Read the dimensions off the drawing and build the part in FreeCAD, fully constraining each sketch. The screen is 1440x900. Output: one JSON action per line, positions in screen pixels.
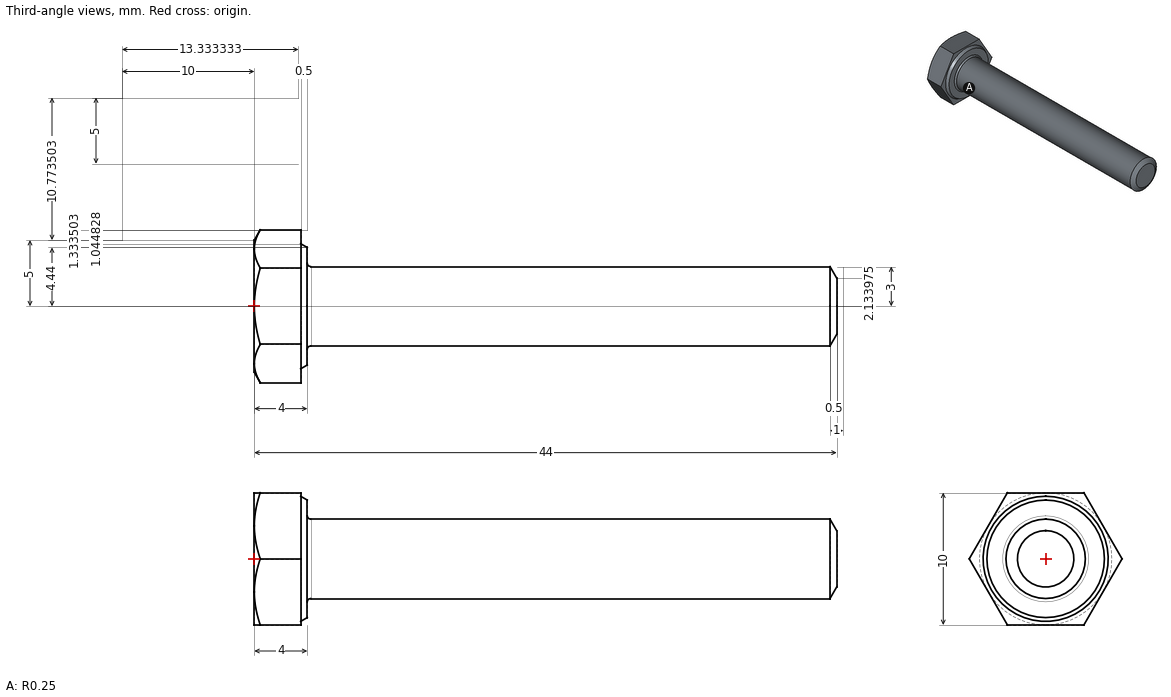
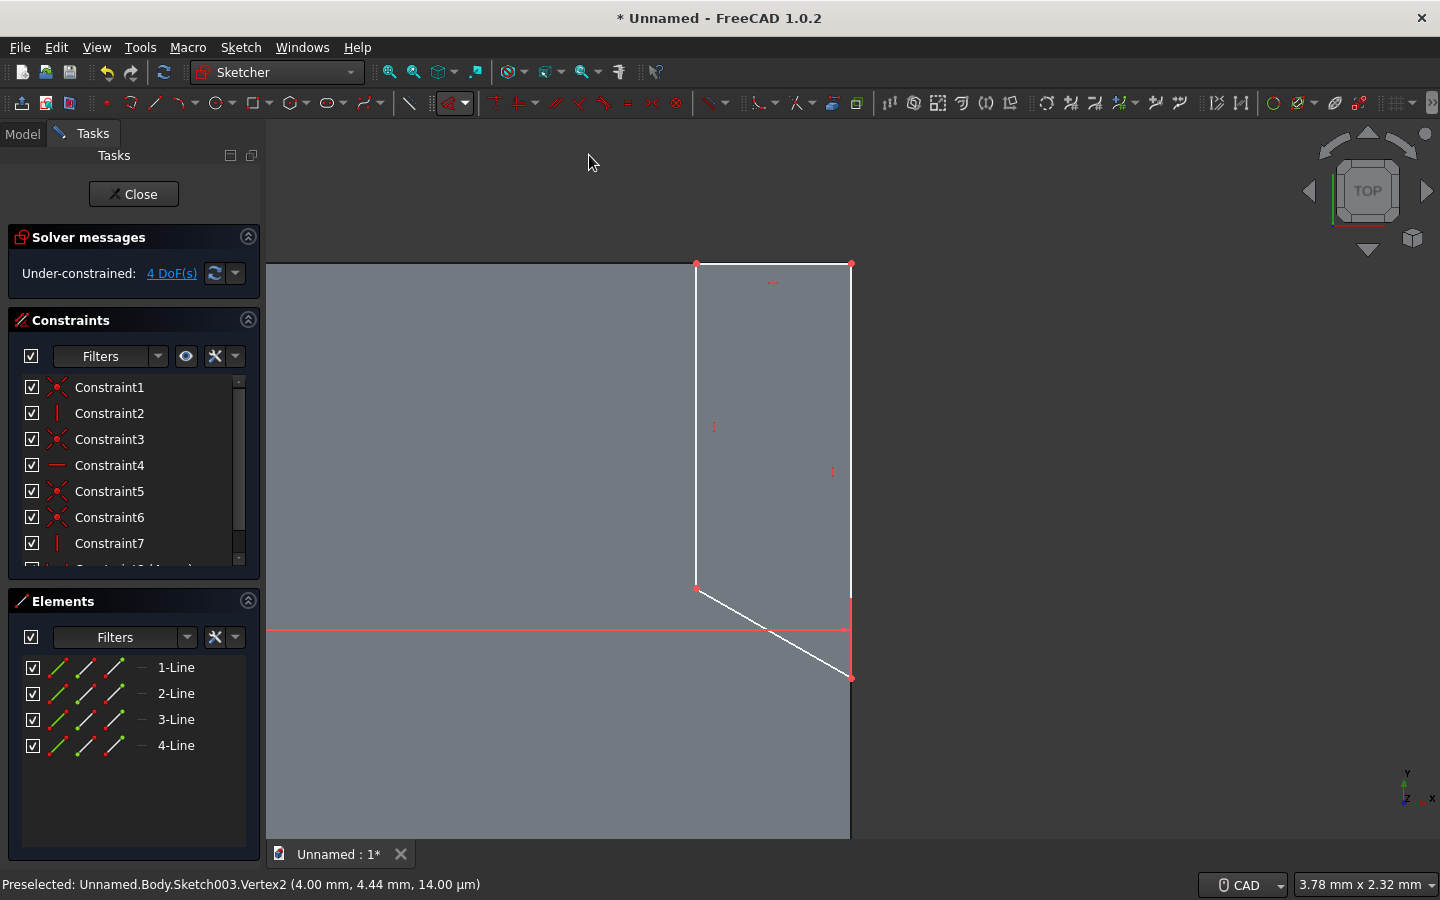
{"action": "left_click", "coordinate": [805, 264]}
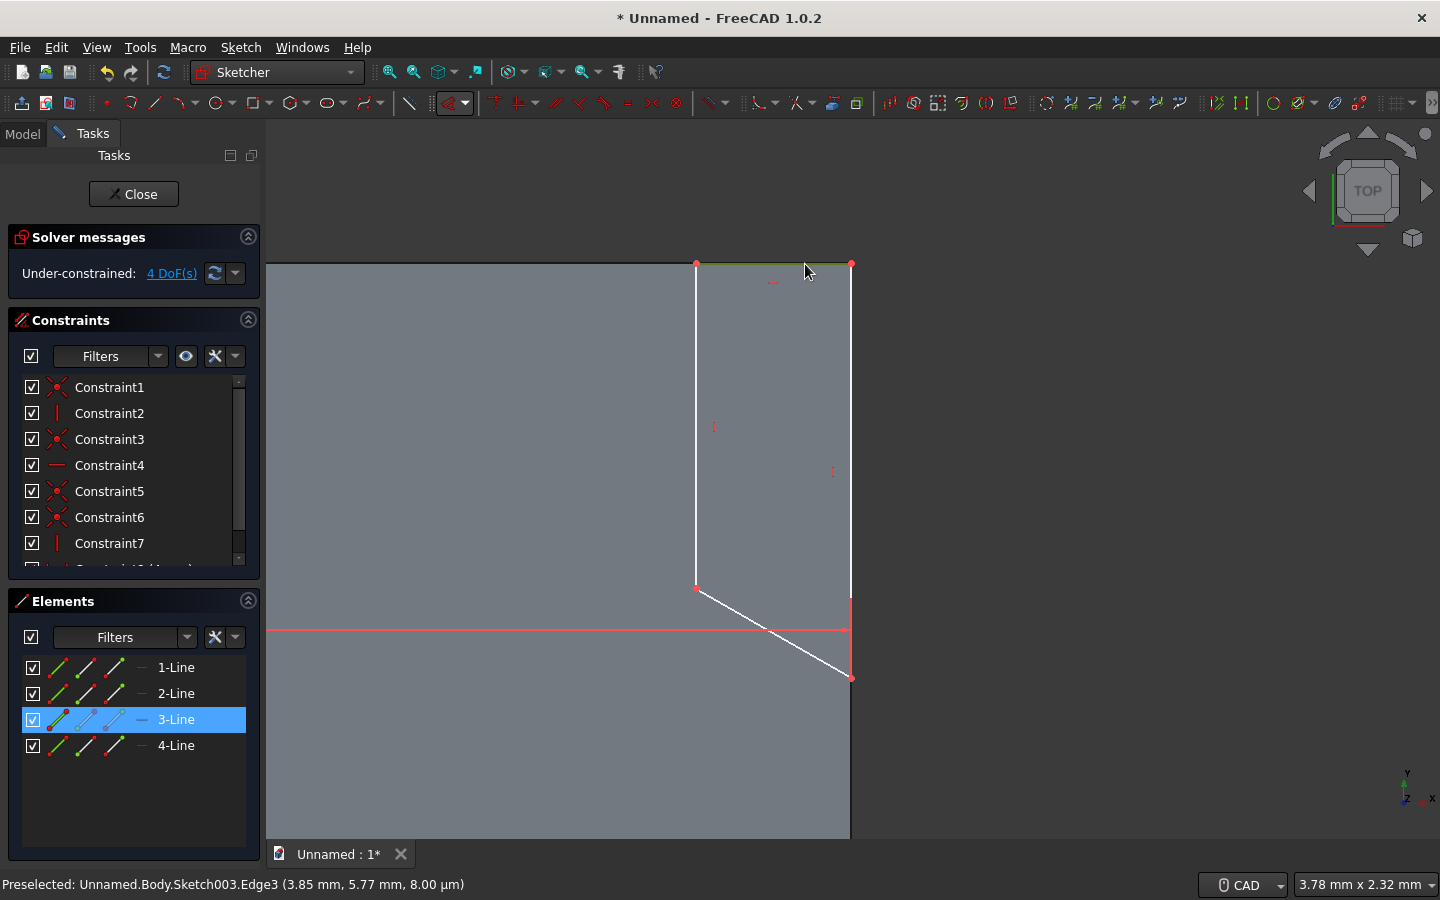
{"action": "left_click", "coordinate": [468, 104]}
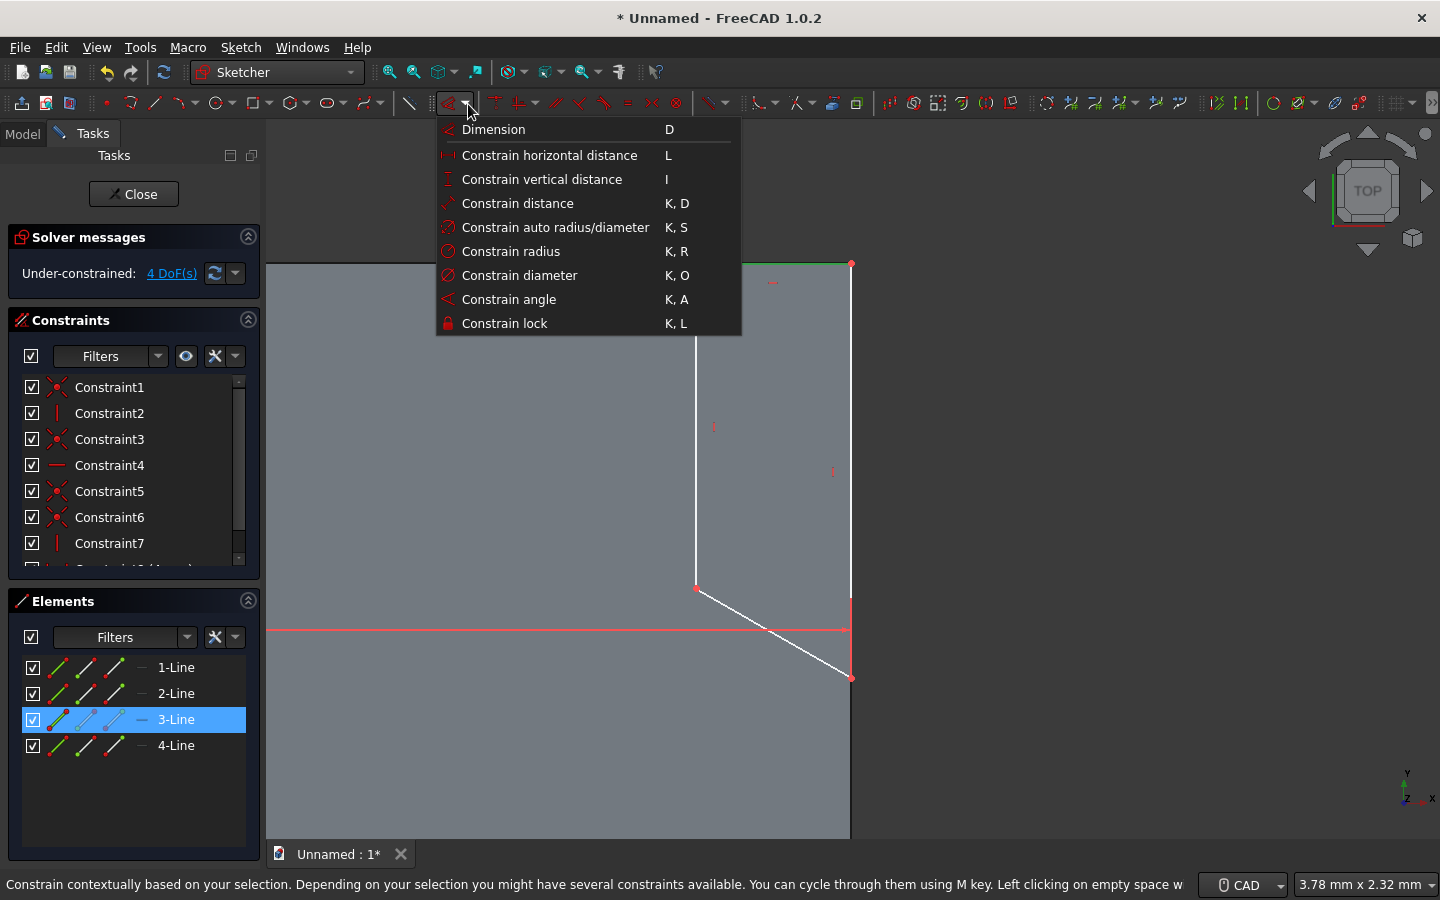
{"action": "left_click", "coordinate": [589, 155]}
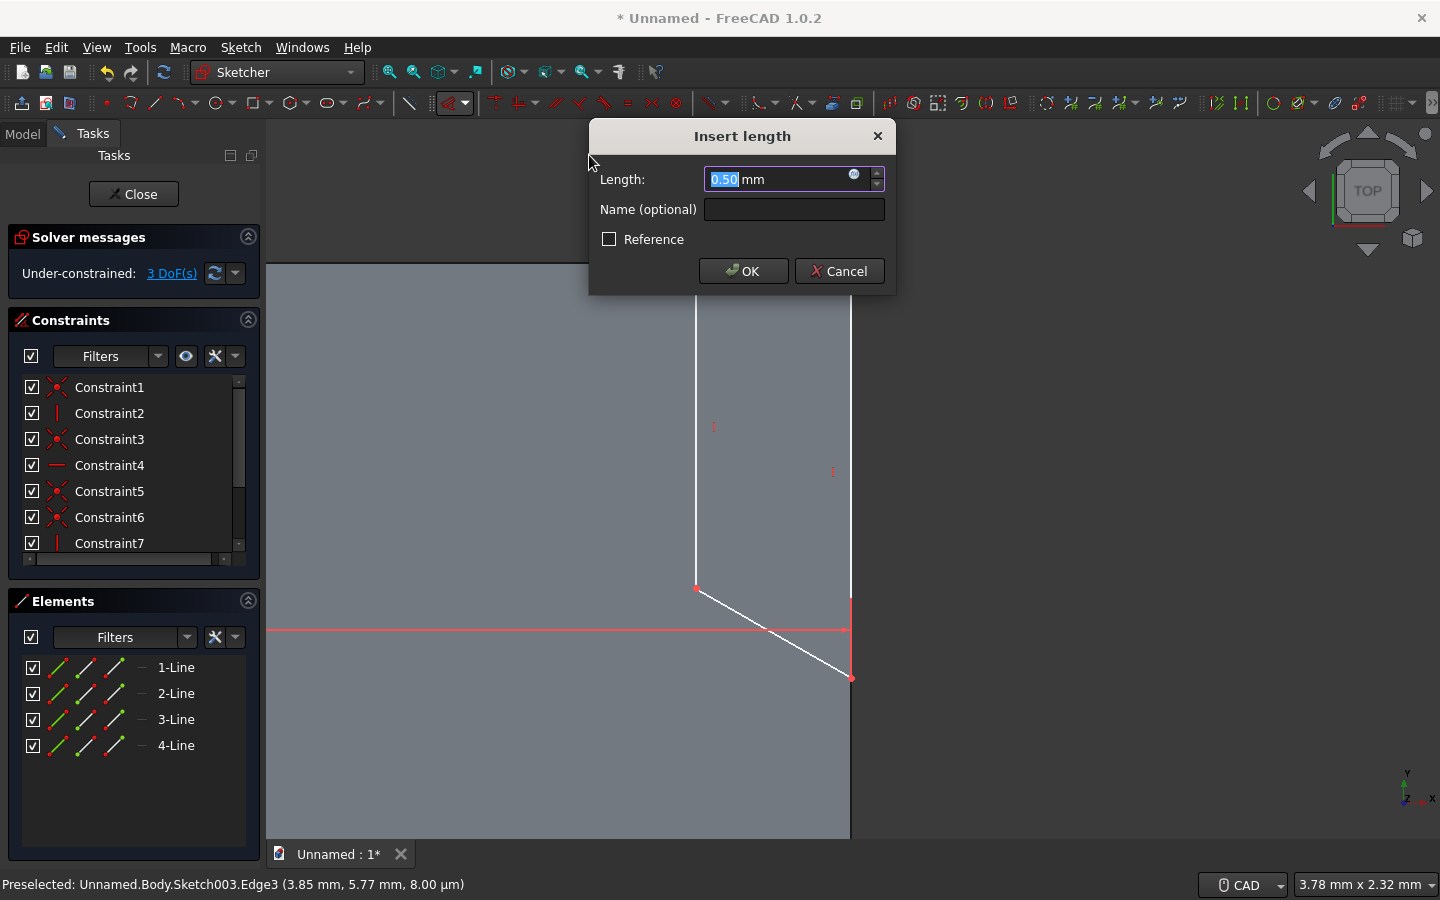
{"action": "type", "text": "0.5"}
{"action": "key", "text": "Return"}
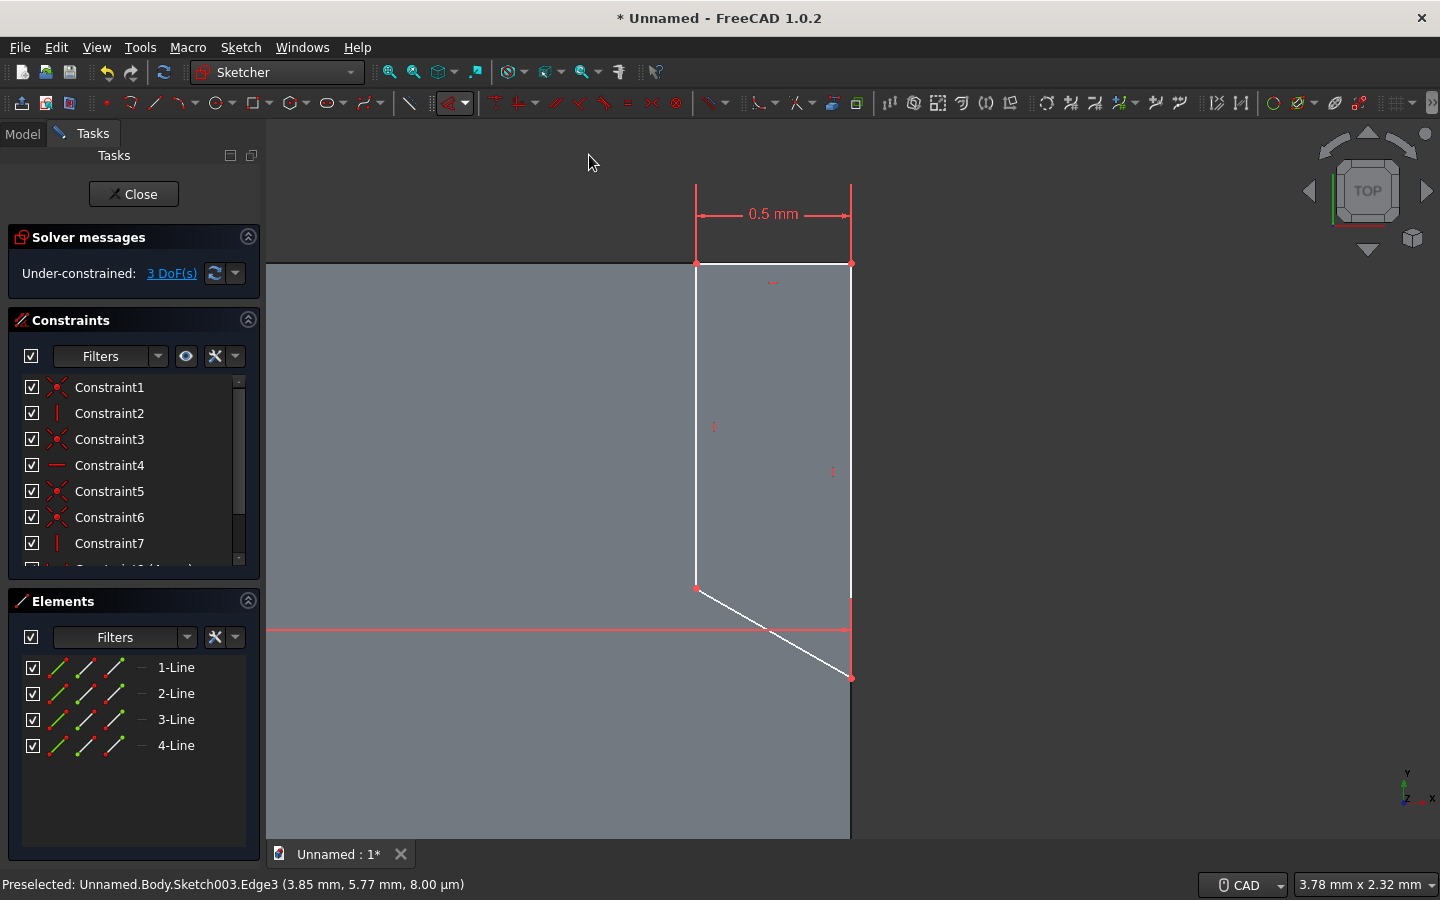
{"action": "left_click", "coordinate": [851, 678]}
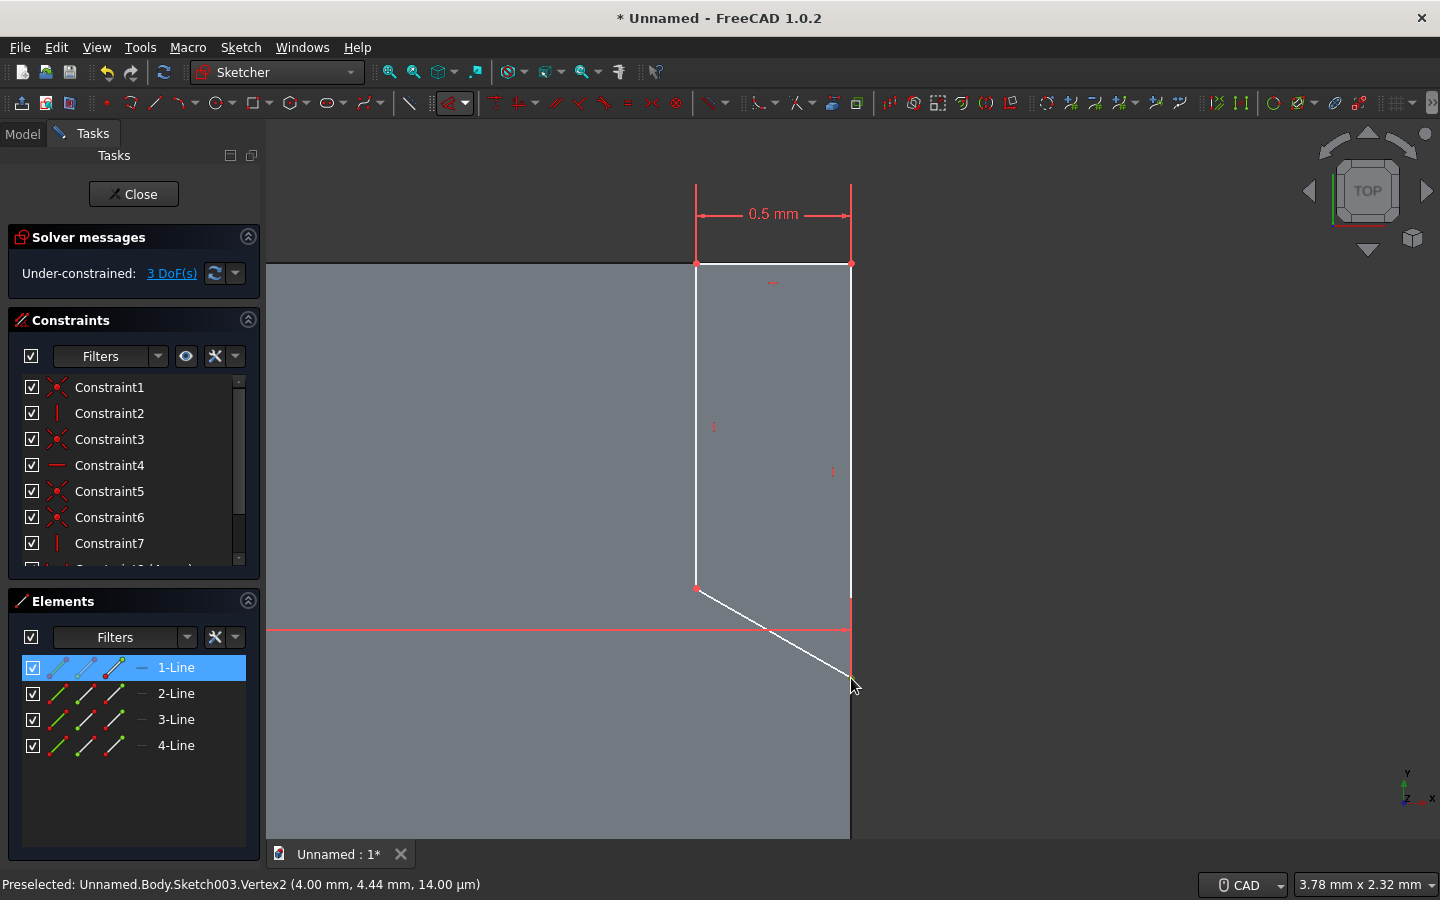
{"action": "key", "text": "i"}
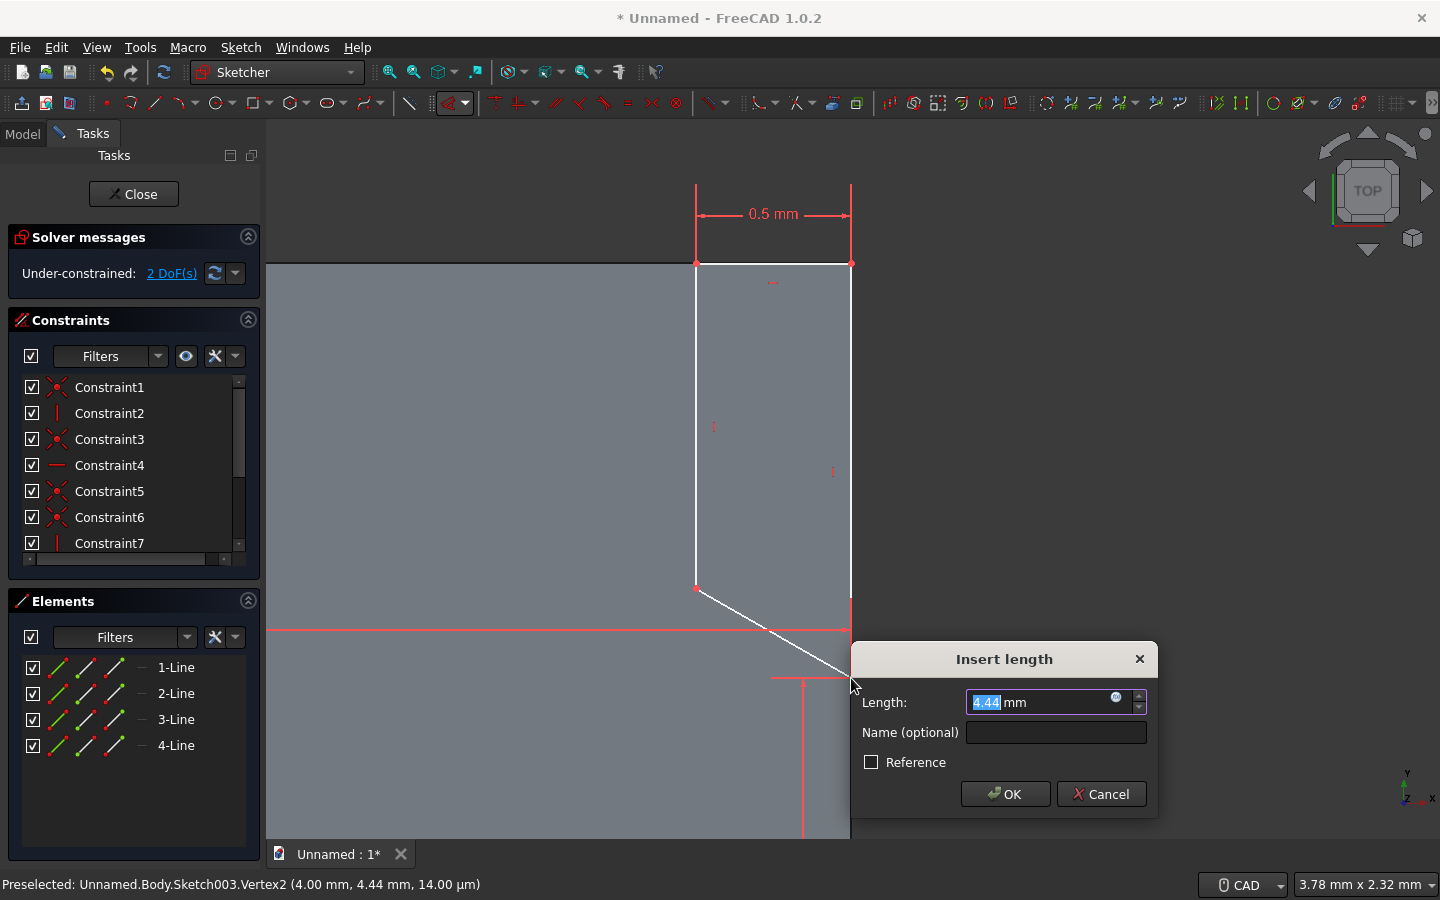
{"action": "type", "text": "4.44"}
{"action": "key", "text": "Return"}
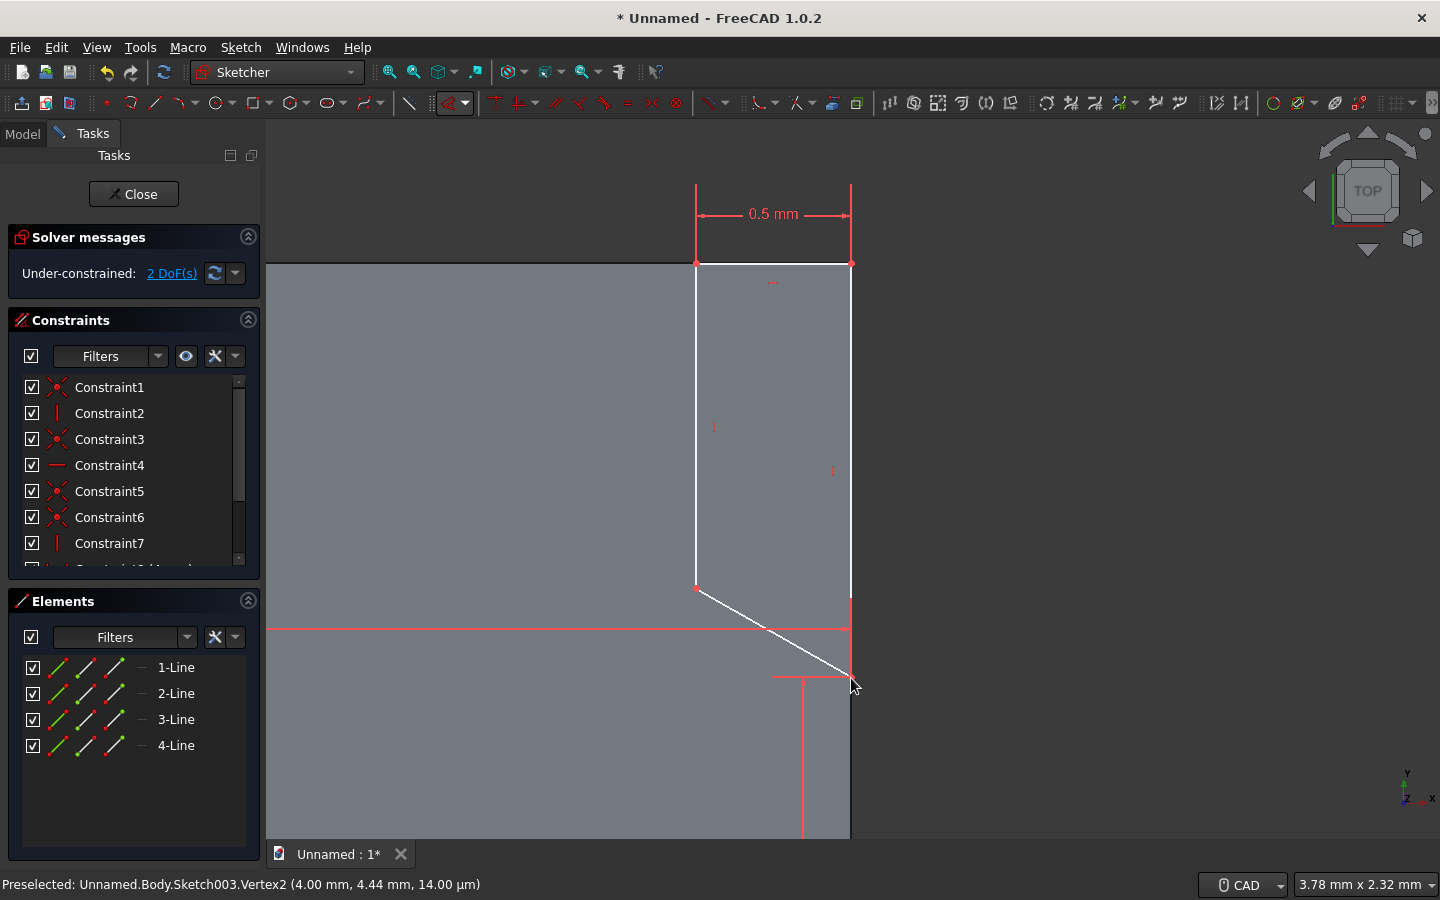
{"action": "left_click", "coordinate": [851, 553]}